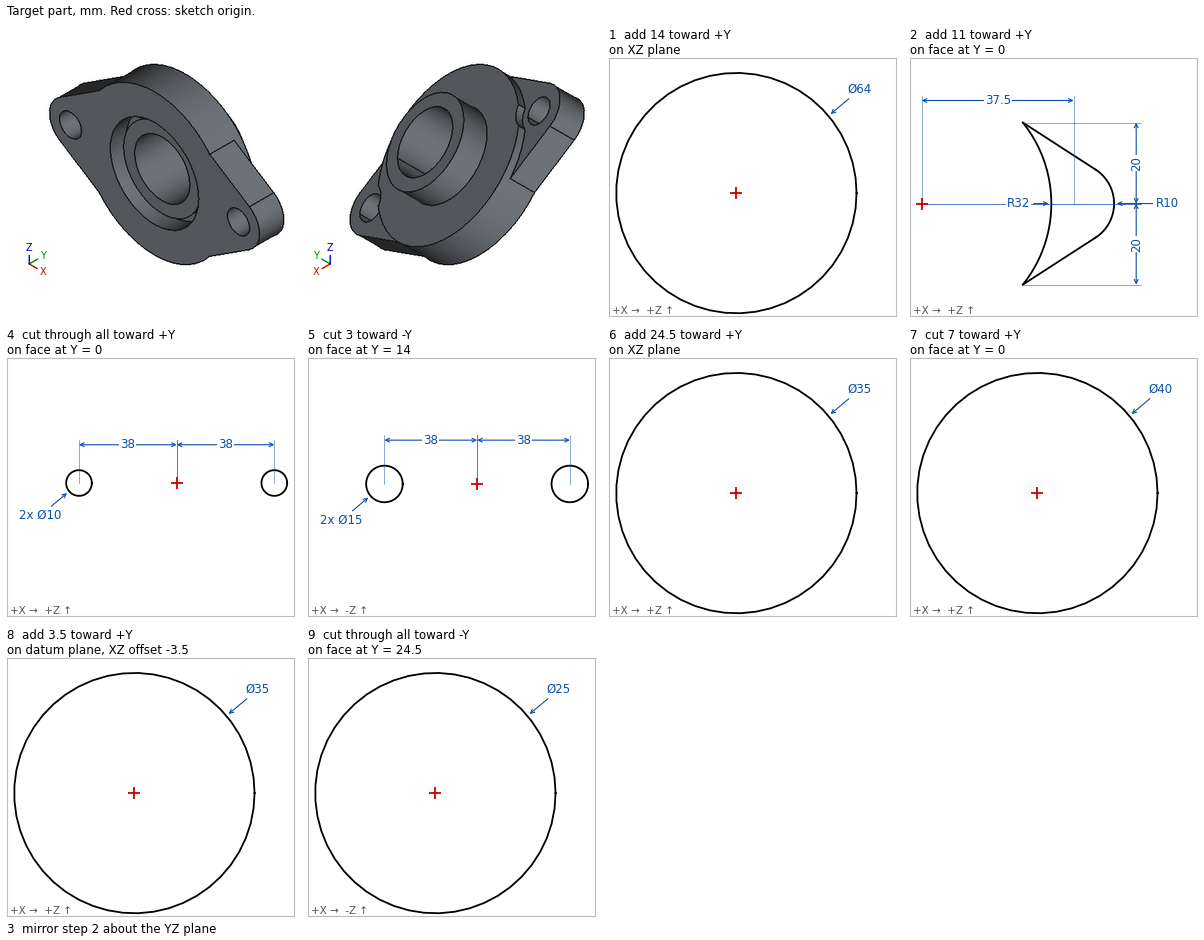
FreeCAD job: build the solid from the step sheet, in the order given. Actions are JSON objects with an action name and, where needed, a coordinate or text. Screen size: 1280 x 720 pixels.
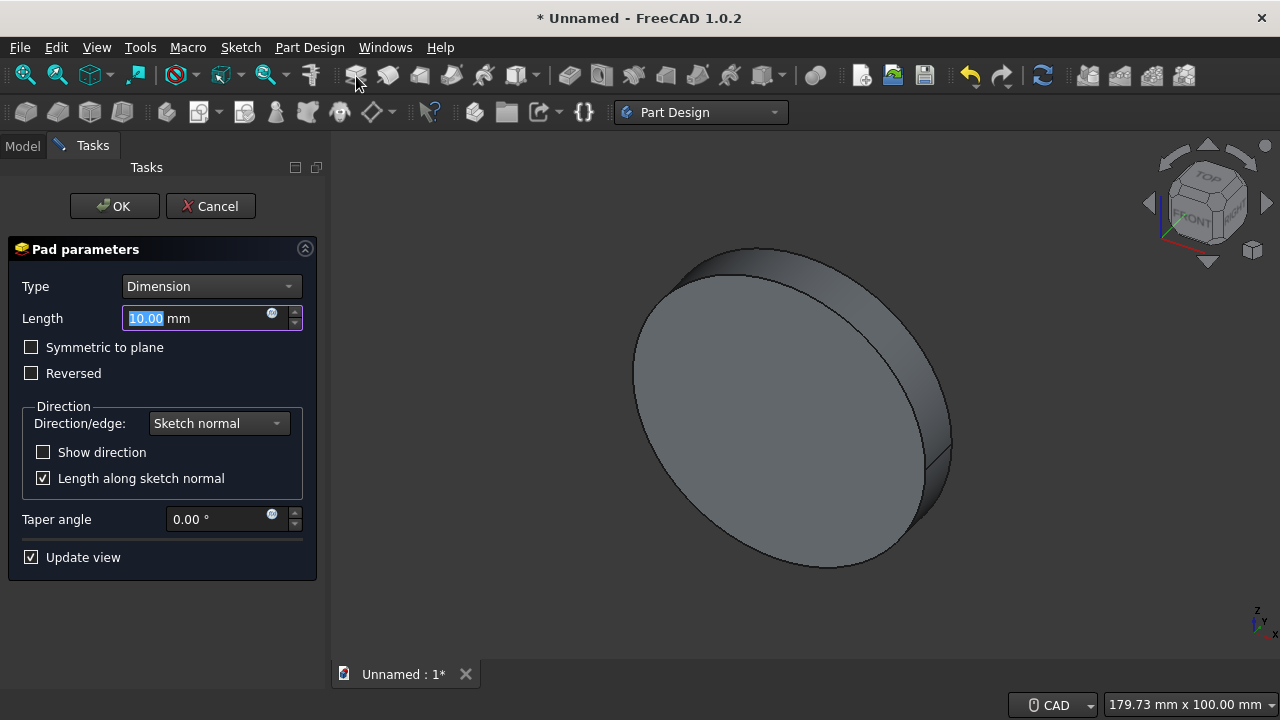
{"action": "type", "text": "14"}
{"action": "key", "text": "Tab"}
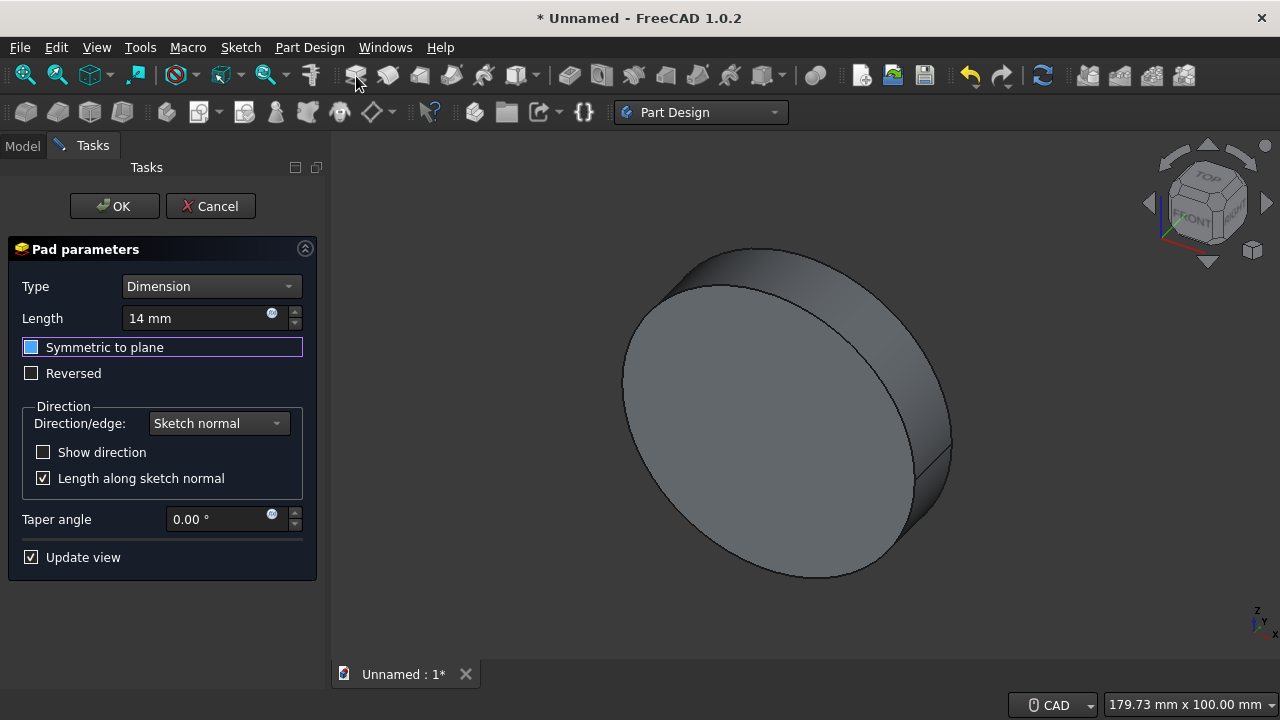
{"action": "left_click", "coordinate": [30, 373]}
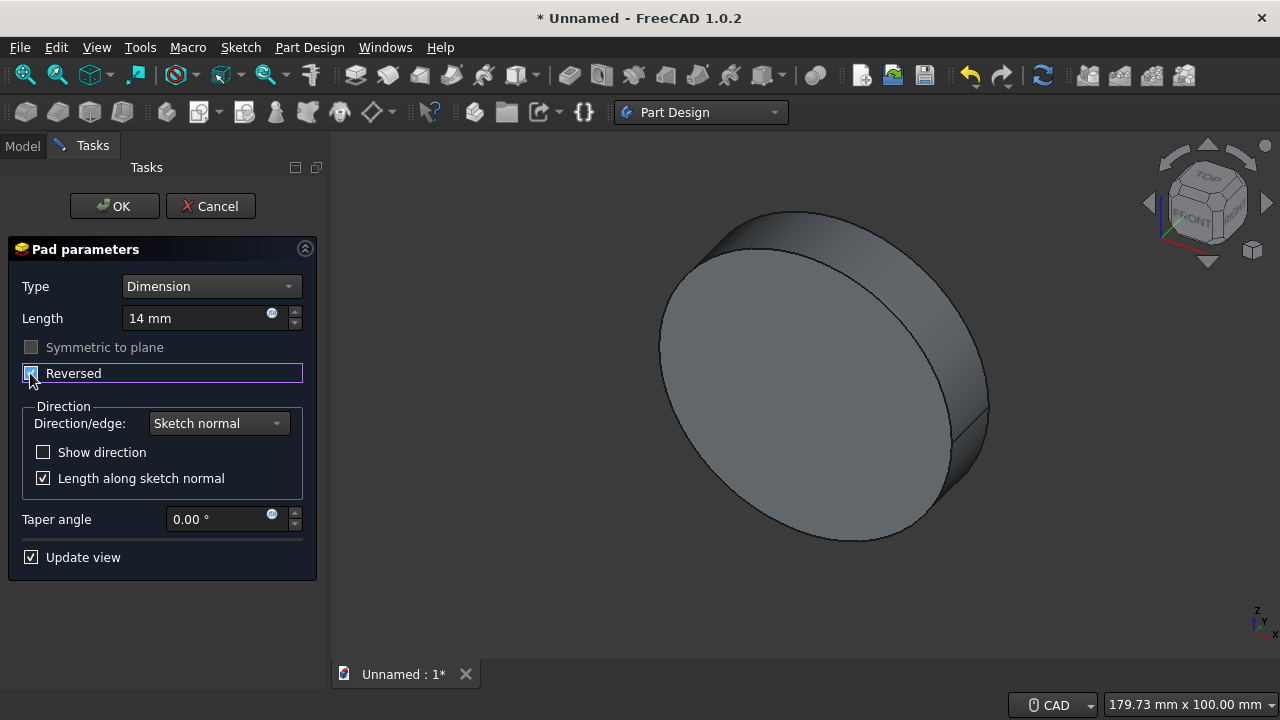
{"action": "left_click", "coordinate": [115, 206]}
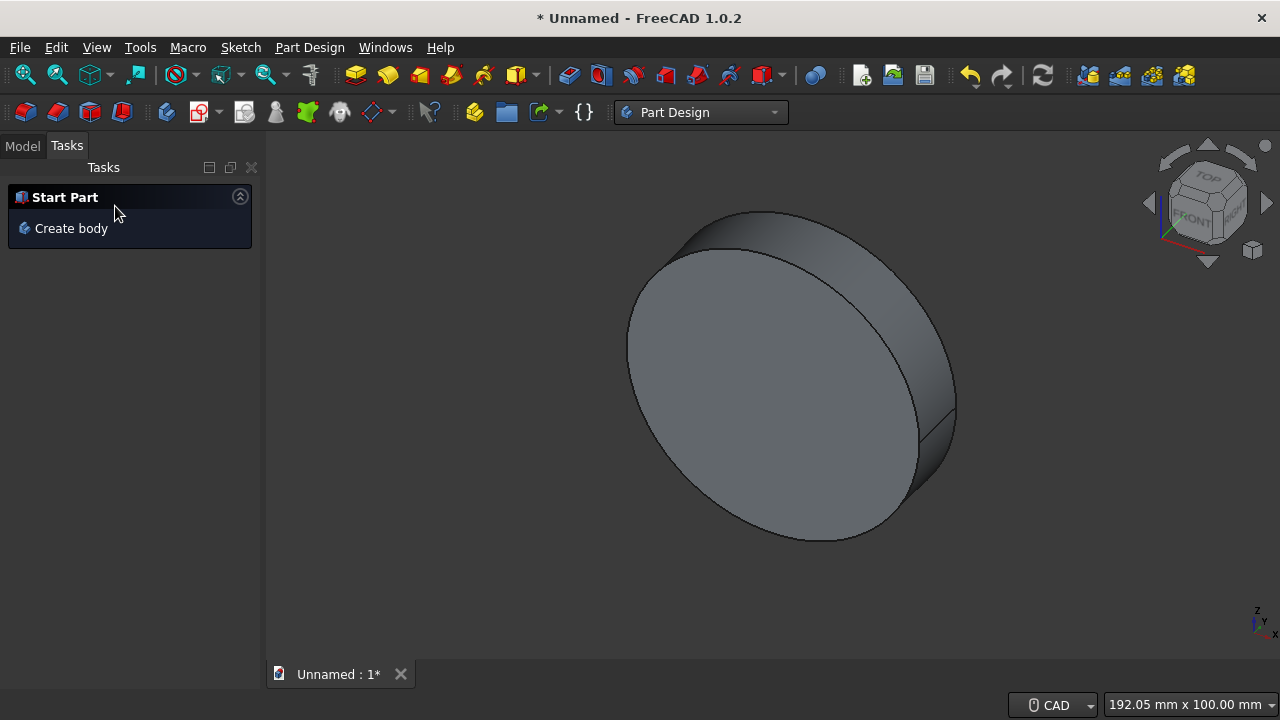
{"action": "left_click", "coordinate": [773, 394]}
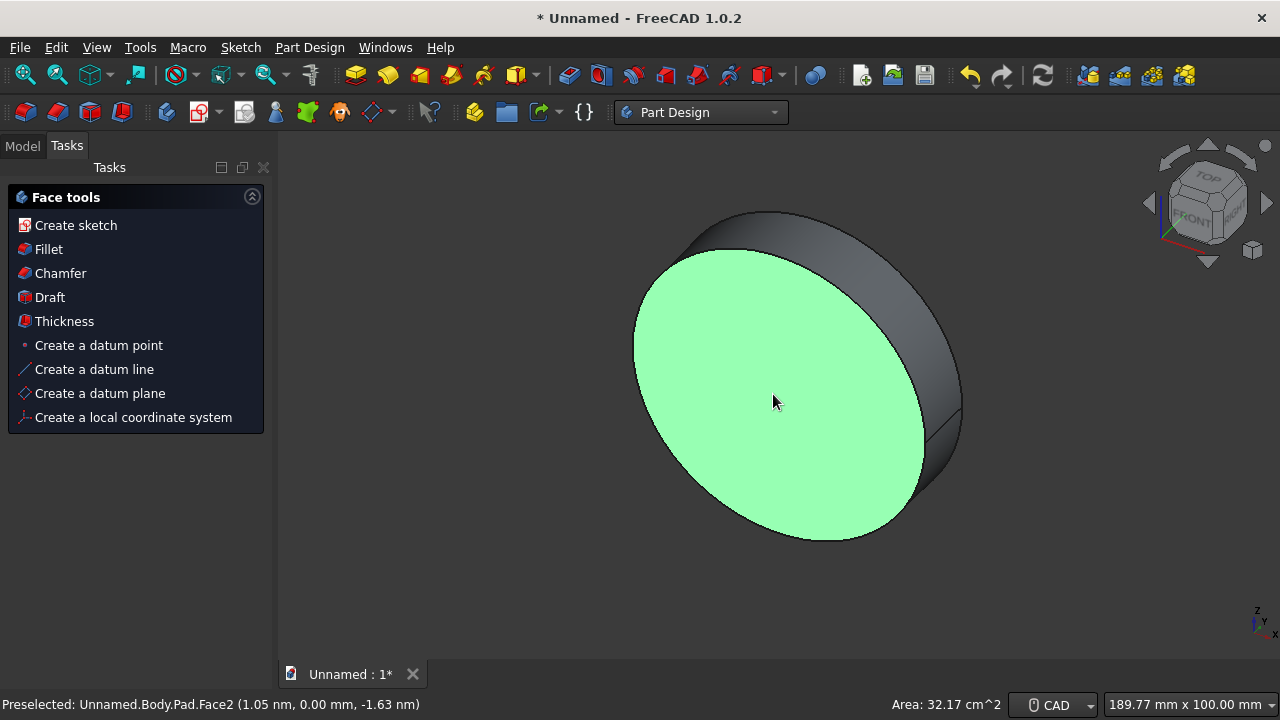
{"action": "left_click", "coordinate": [200, 112]}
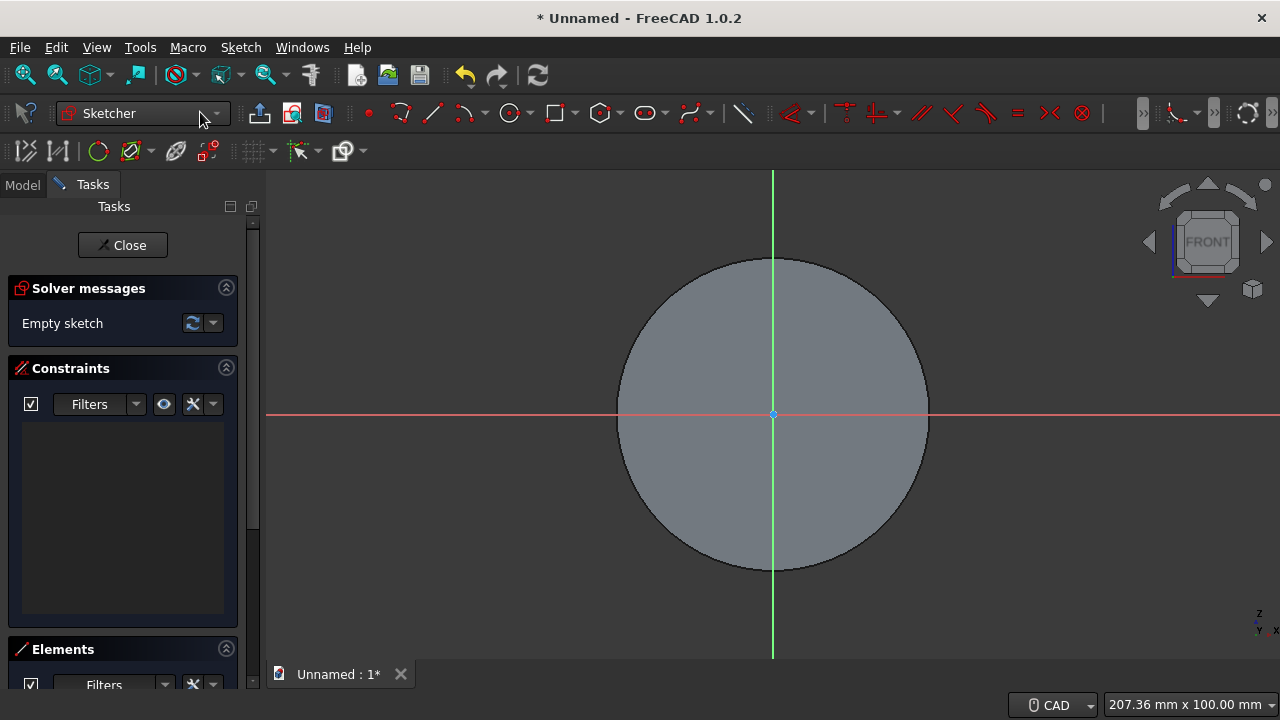
{"action": "scroll", "coordinate": [1115, 414], "scroll_direction": "up", "scroll_amount": 2}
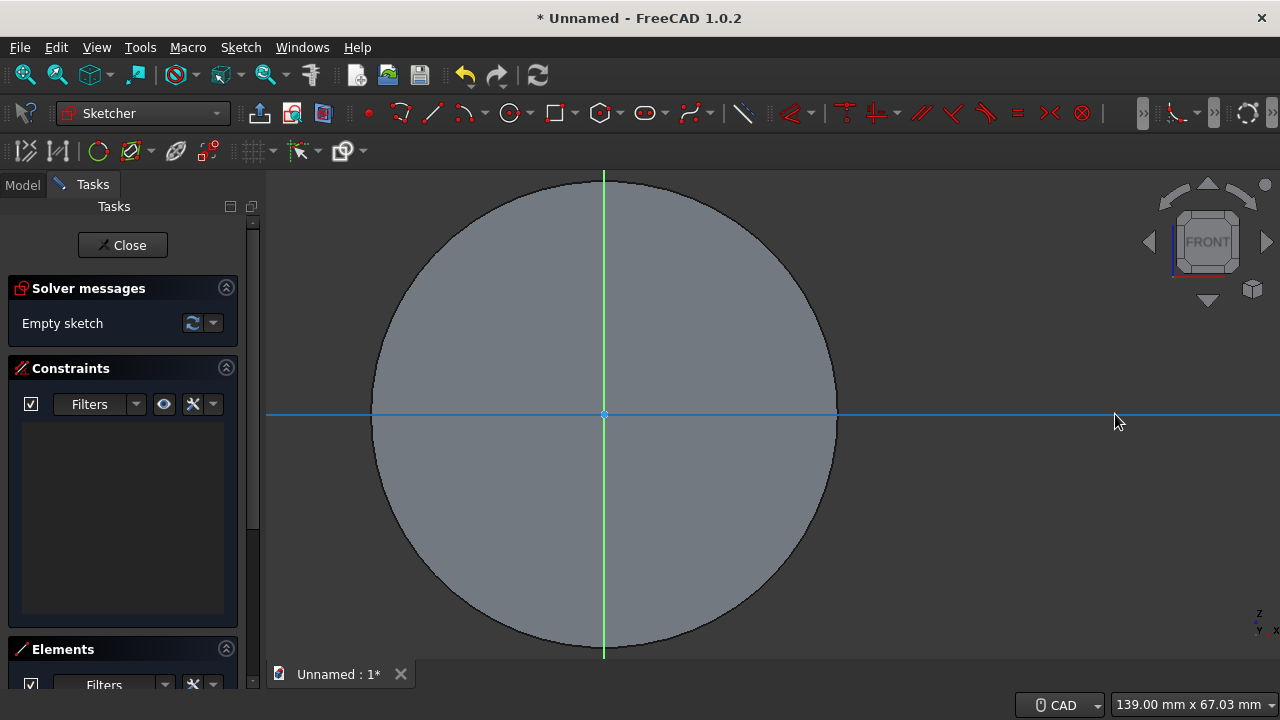
{"action": "left_click", "coordinate": [434, 114]}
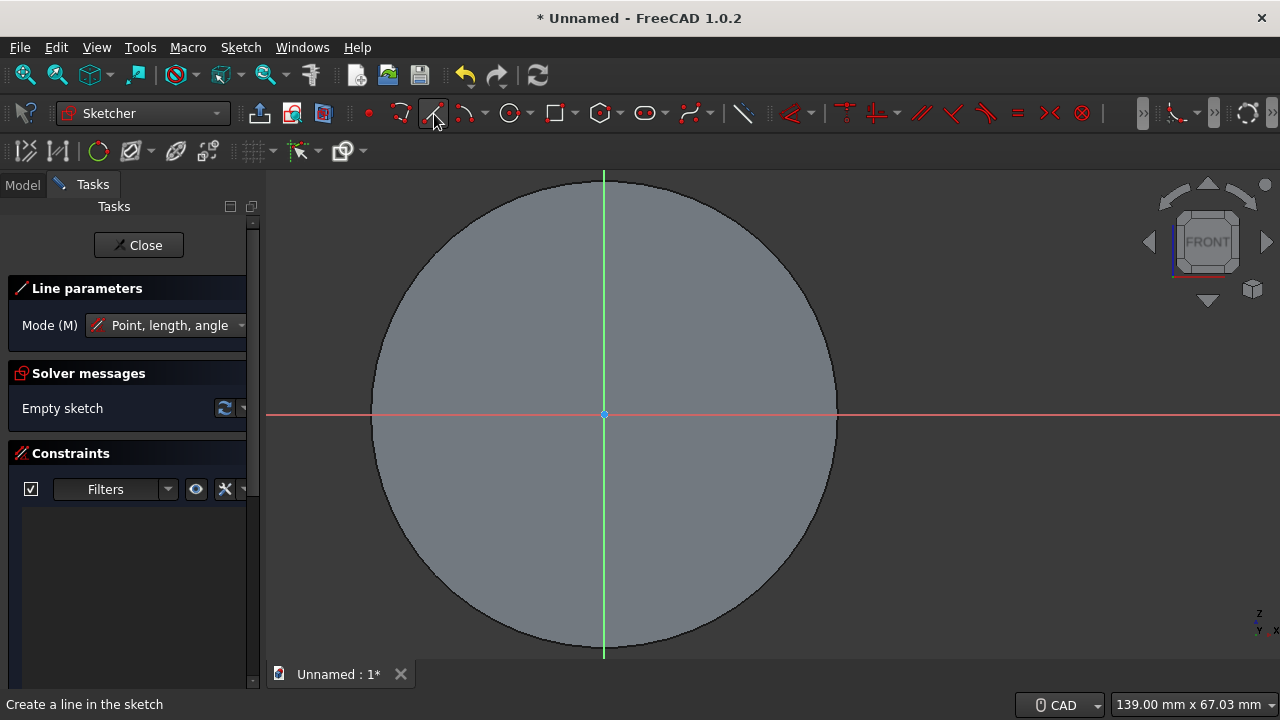
{"action": "left_click", "coordinate": [918, 476]}
{"action": "left_click", "coordinate": [787, 560]}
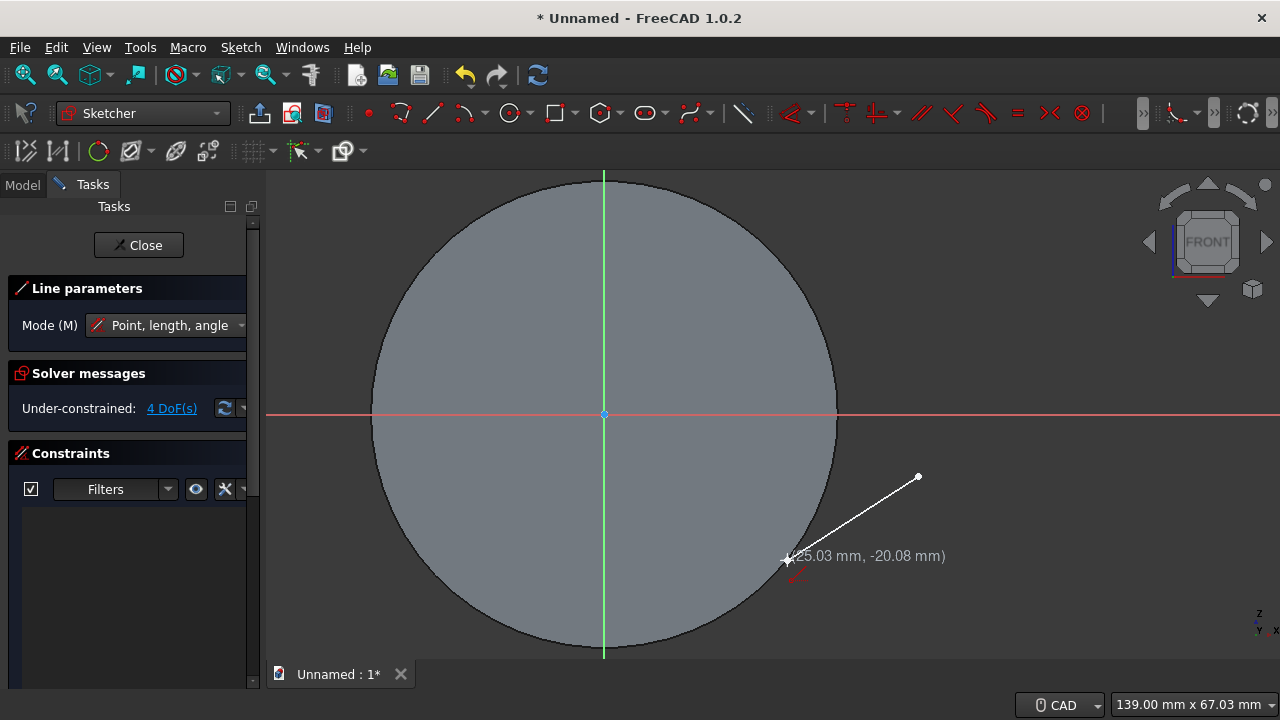
{"action": "left_click", "coordinate": [787, 269]}
{"action": "left_click", "coordinate": [918, 353]}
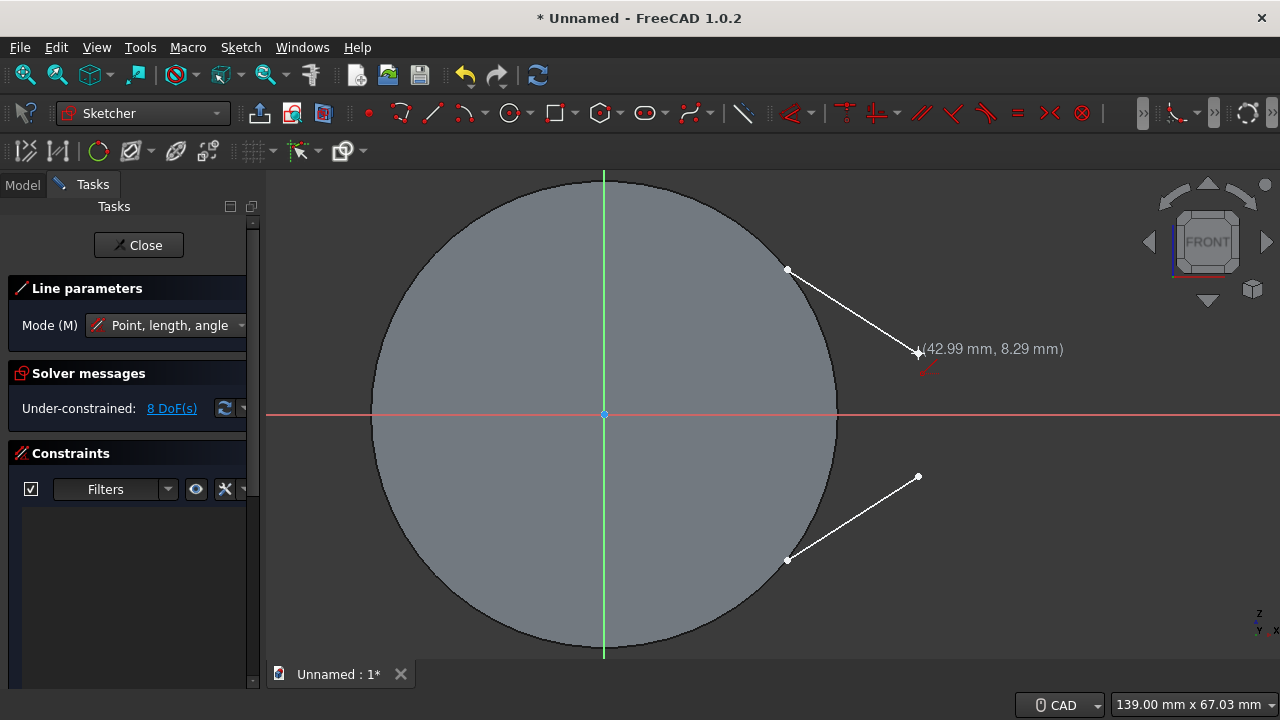
{"action": "key", "text": "g 3 a"}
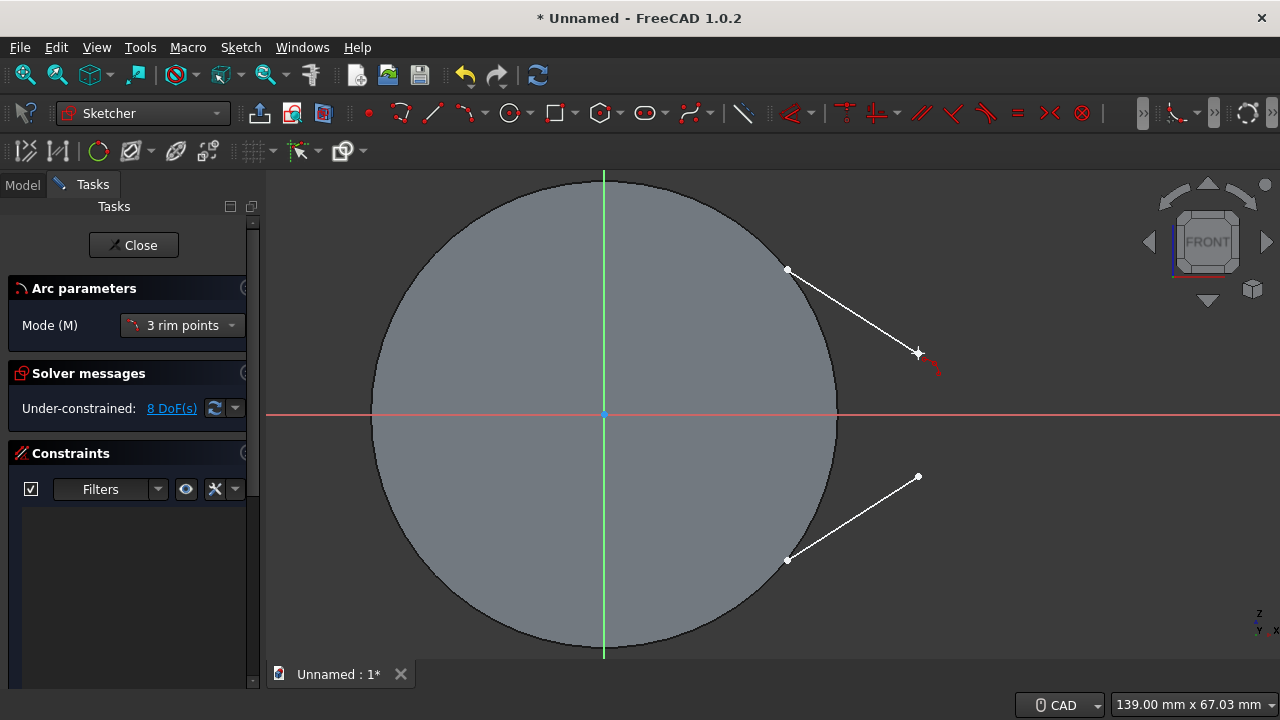
{"action": "left_click", "coordinate": [787, 561]}
{"action": "left_click", "coordinate": [787, 270]}
{"action": "left_click", "coordinate": [836, 446]}